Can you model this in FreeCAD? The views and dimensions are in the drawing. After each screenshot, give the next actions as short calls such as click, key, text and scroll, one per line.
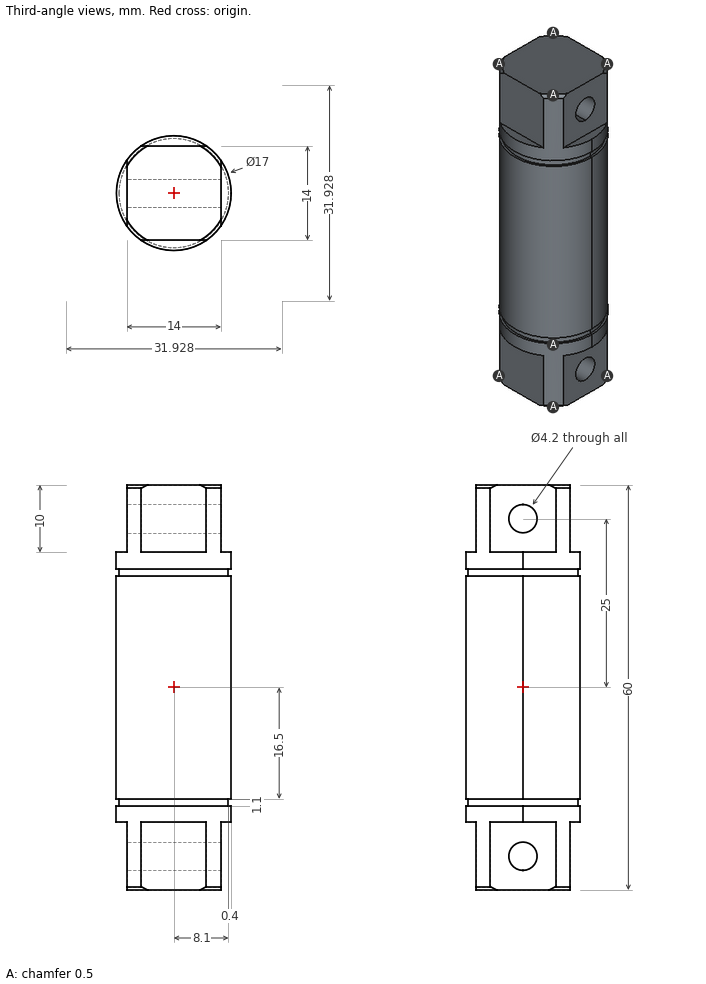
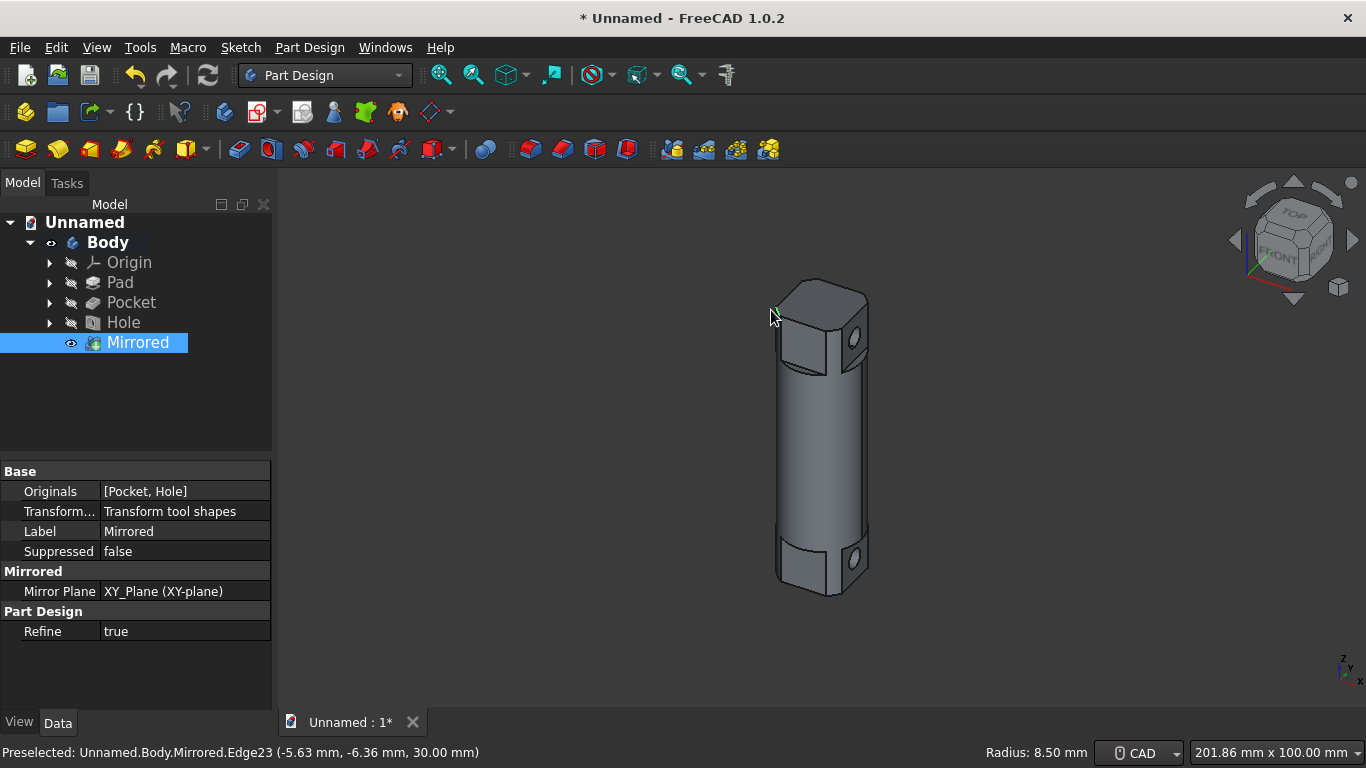
click(834, 329, ctrl)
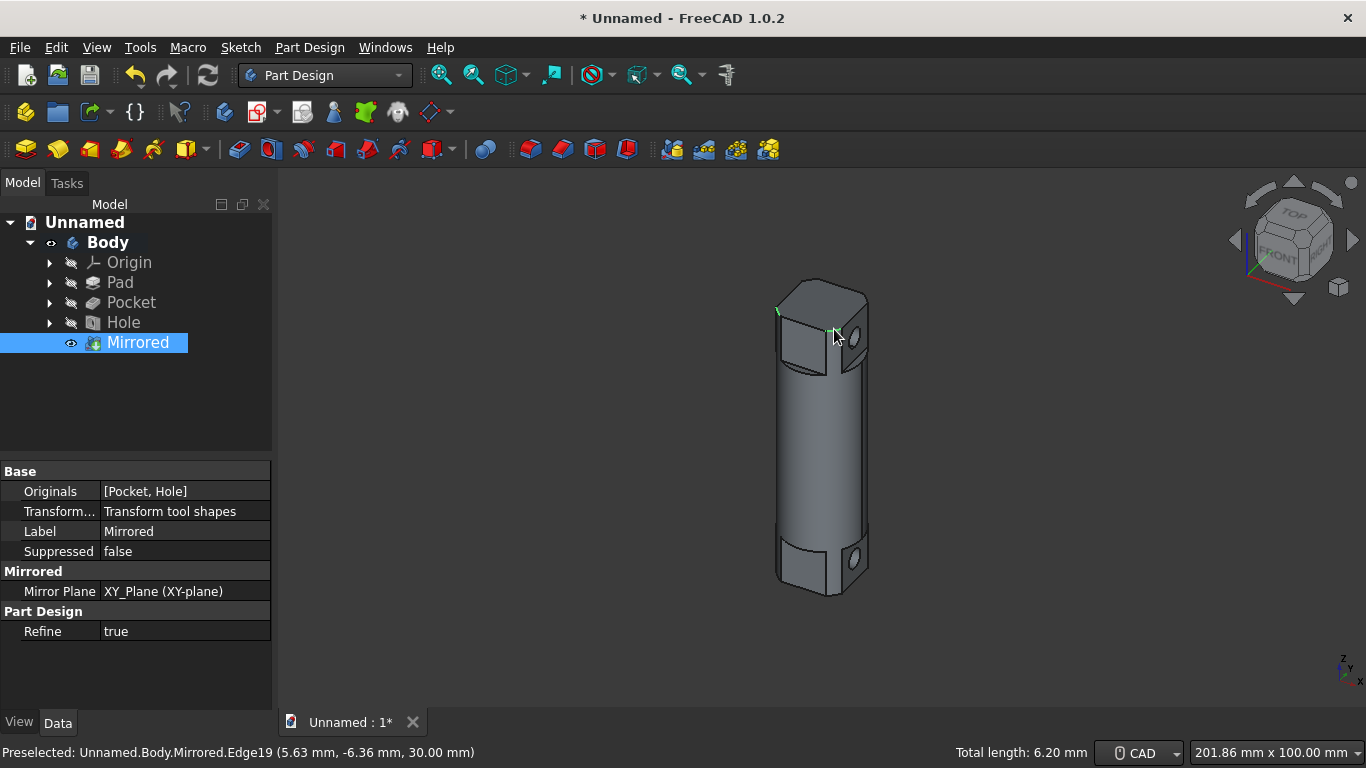
scroll(866, 562, up, 5)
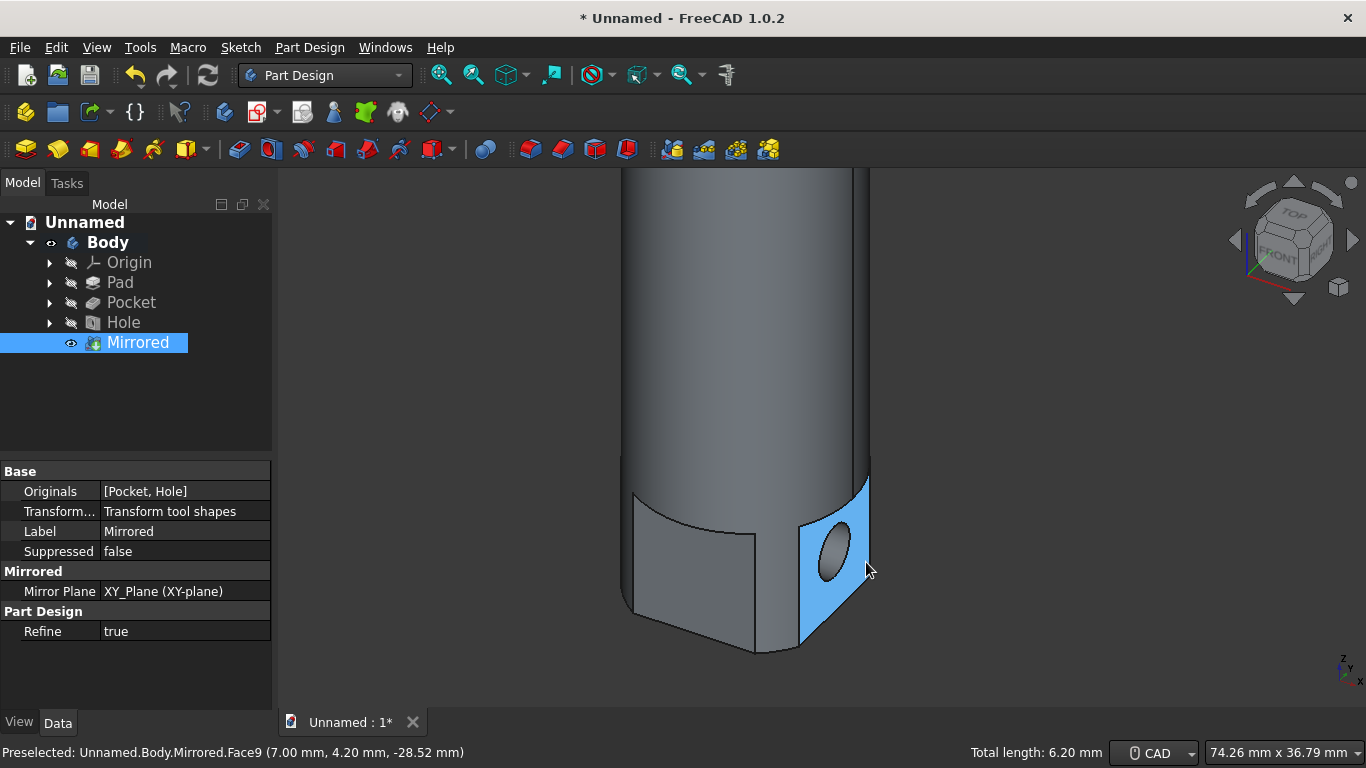
click(442, 76)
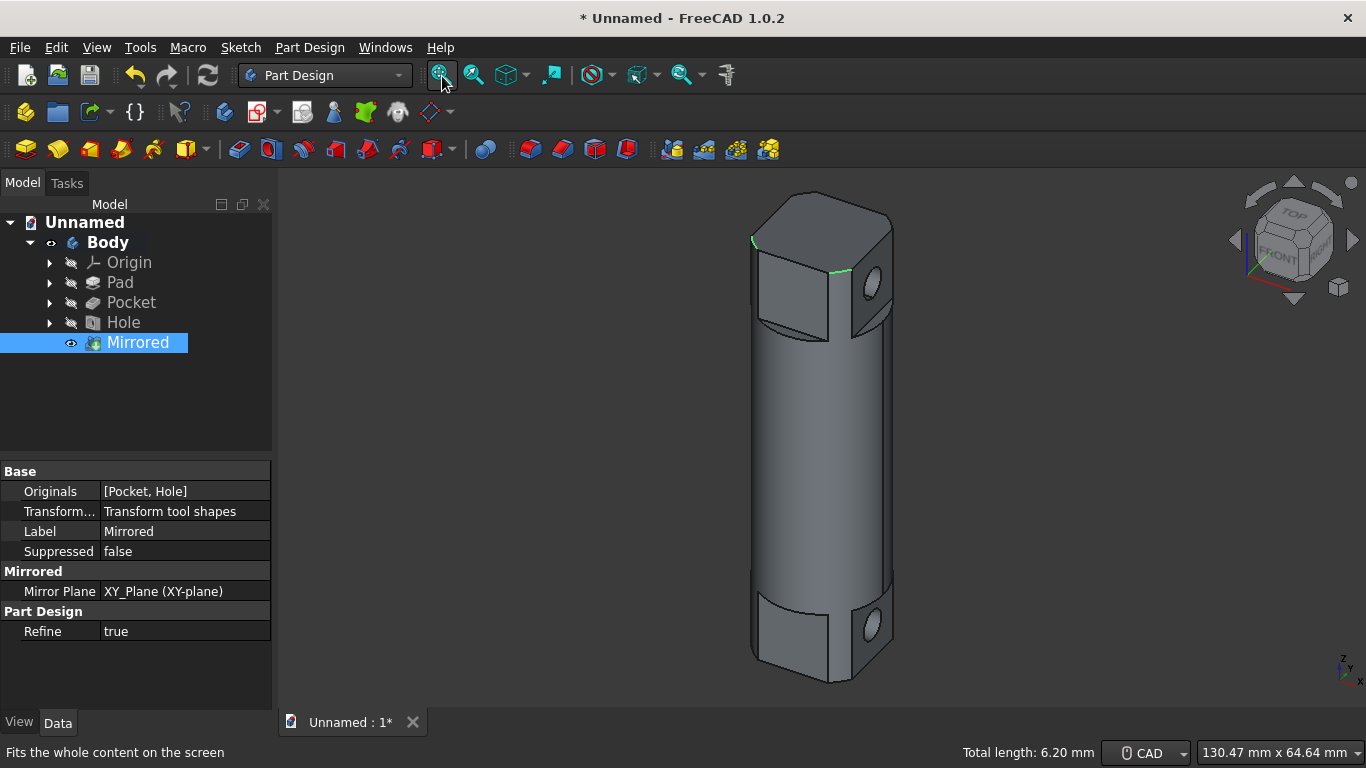
click(891, 222, ctrl)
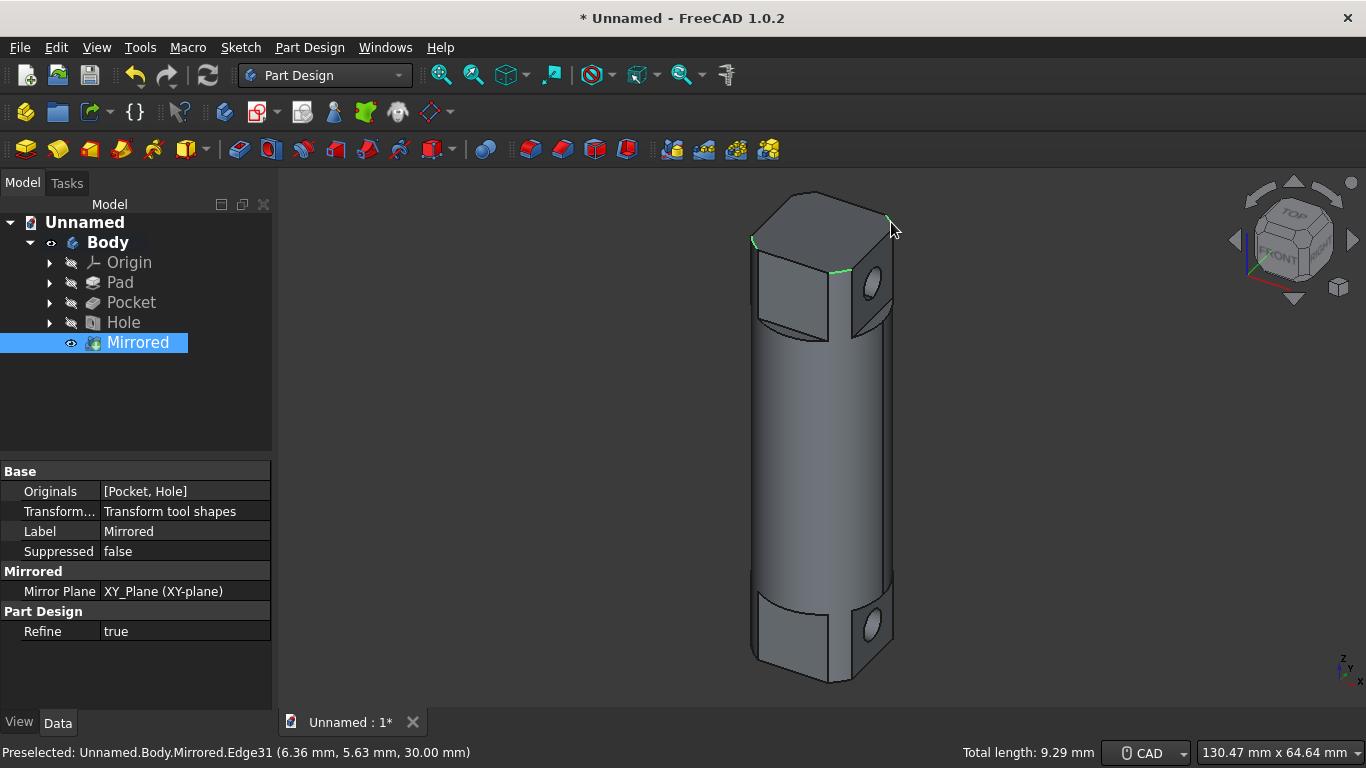
key(v)
key(f)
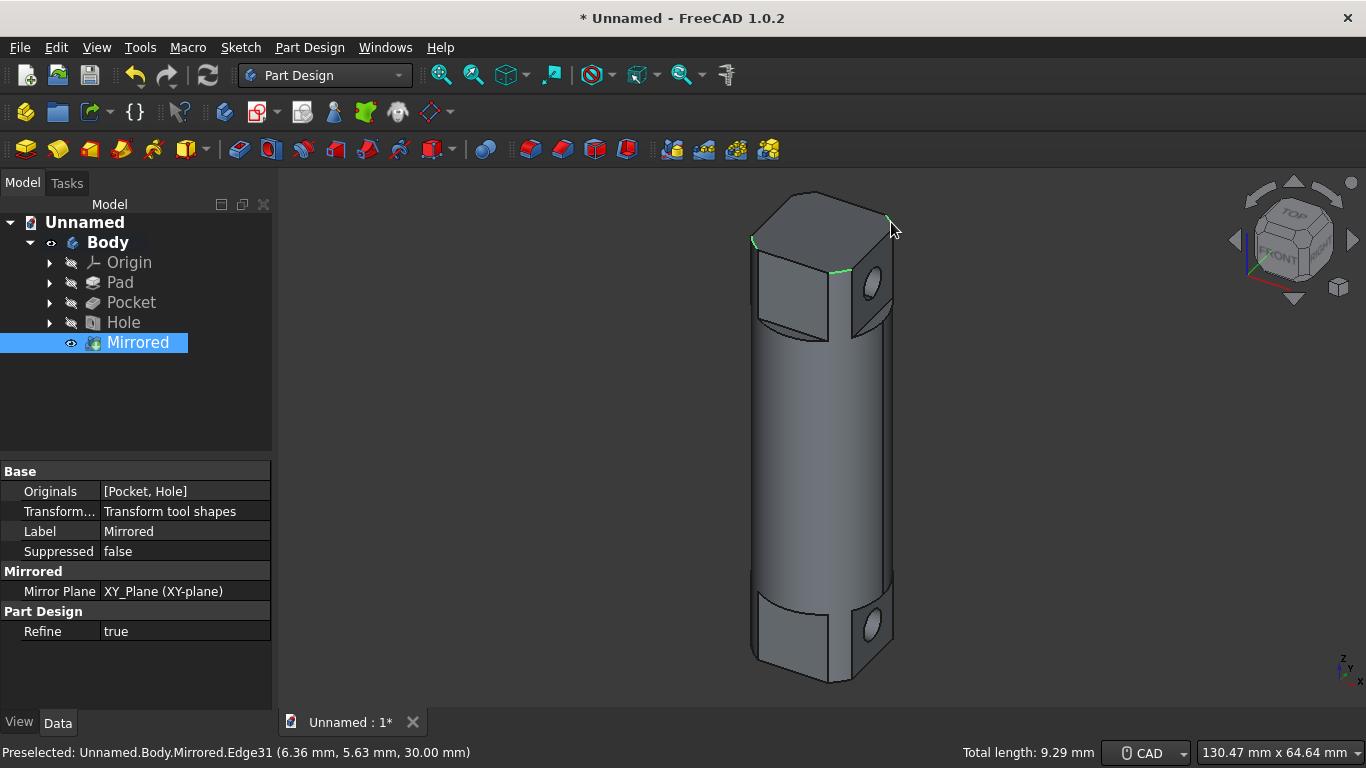
key(0)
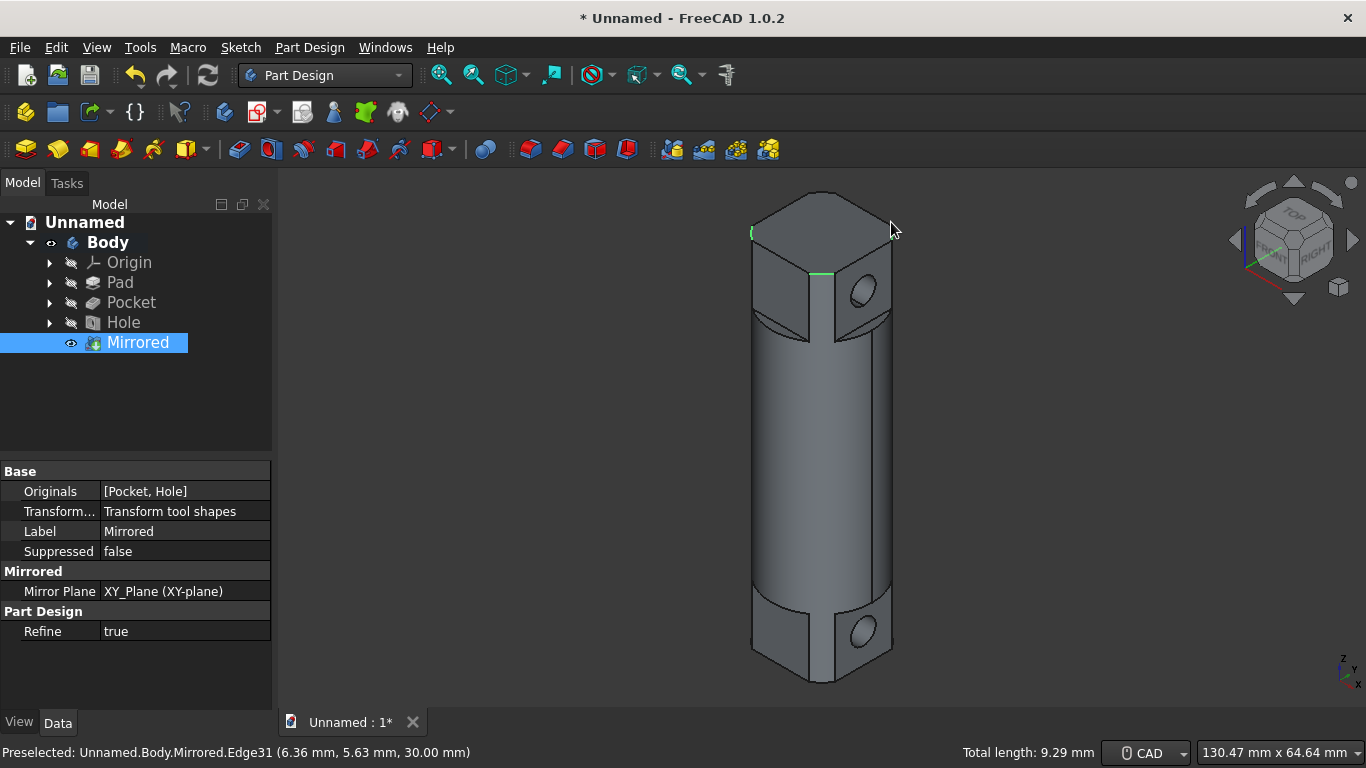
key(2)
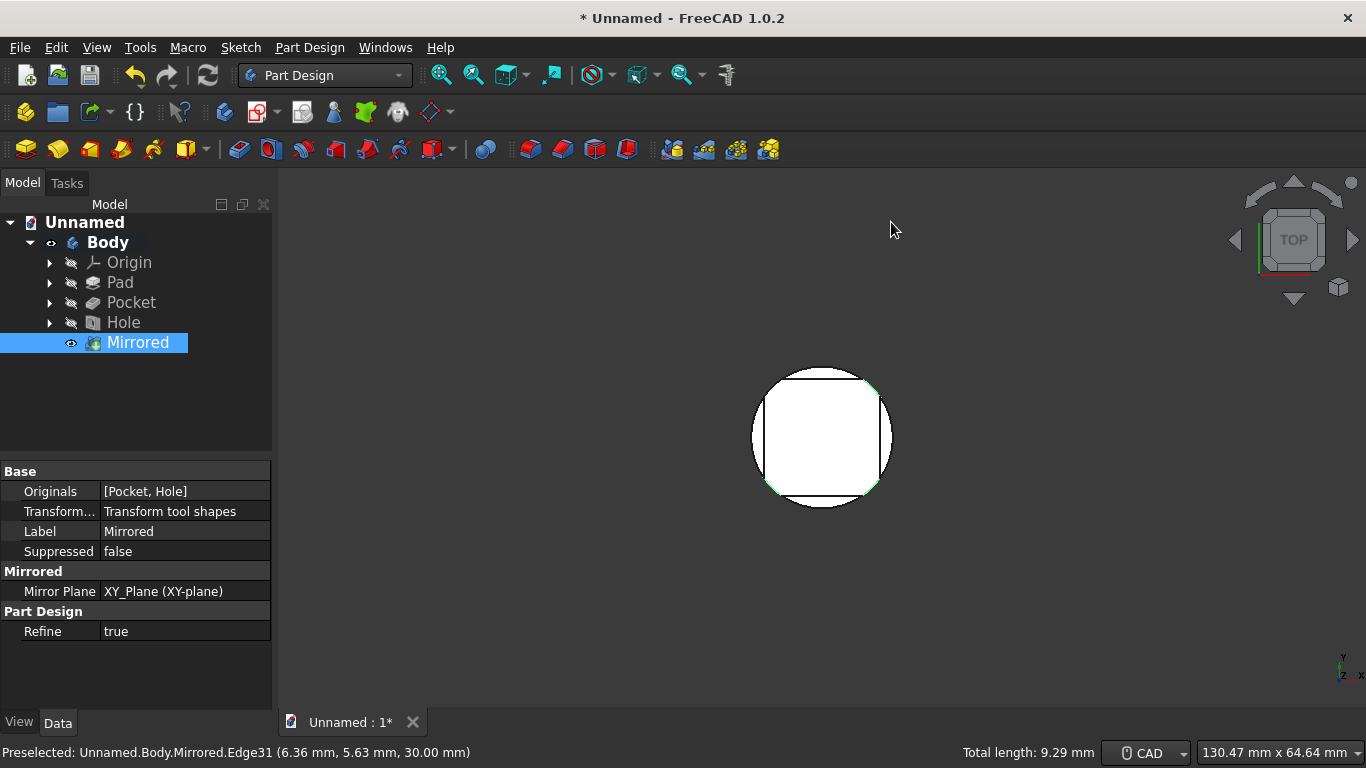
key(v)
key(f)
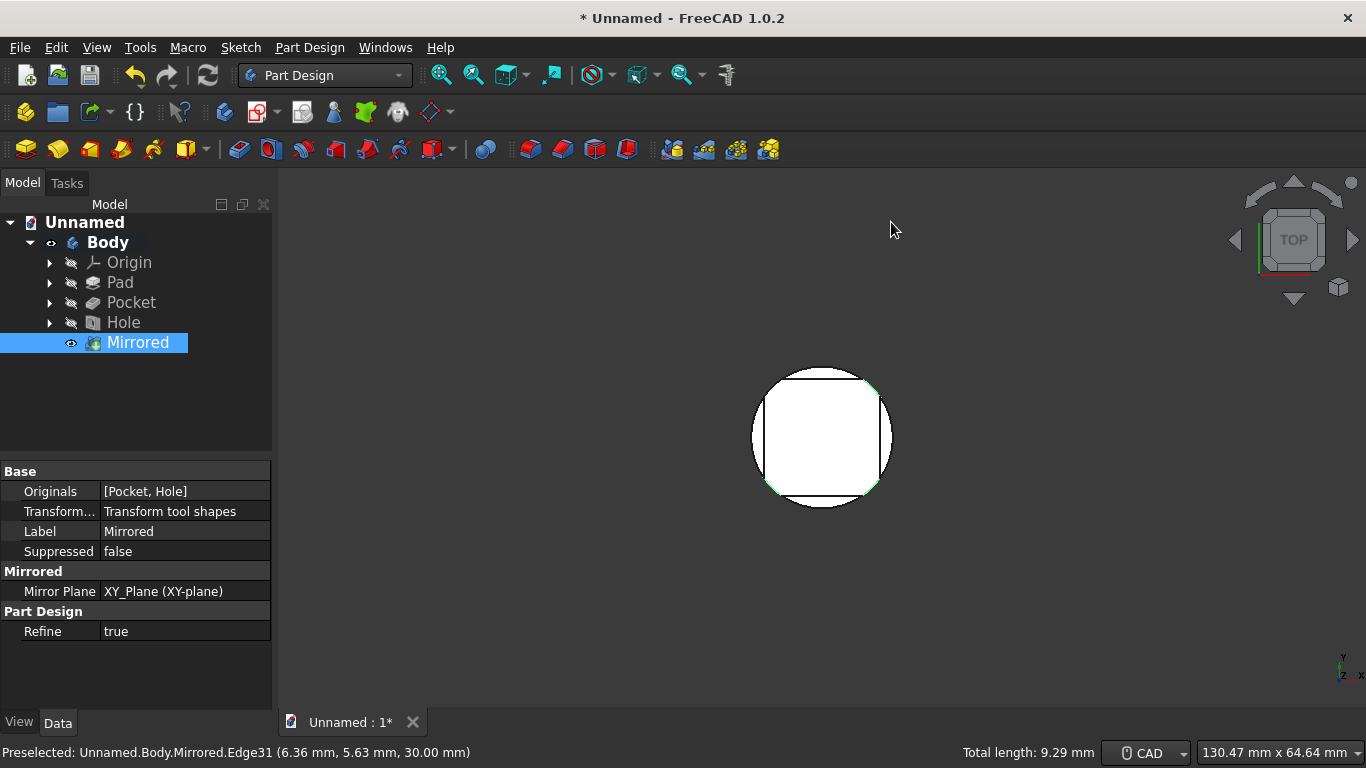
click(772, 386, ctrl)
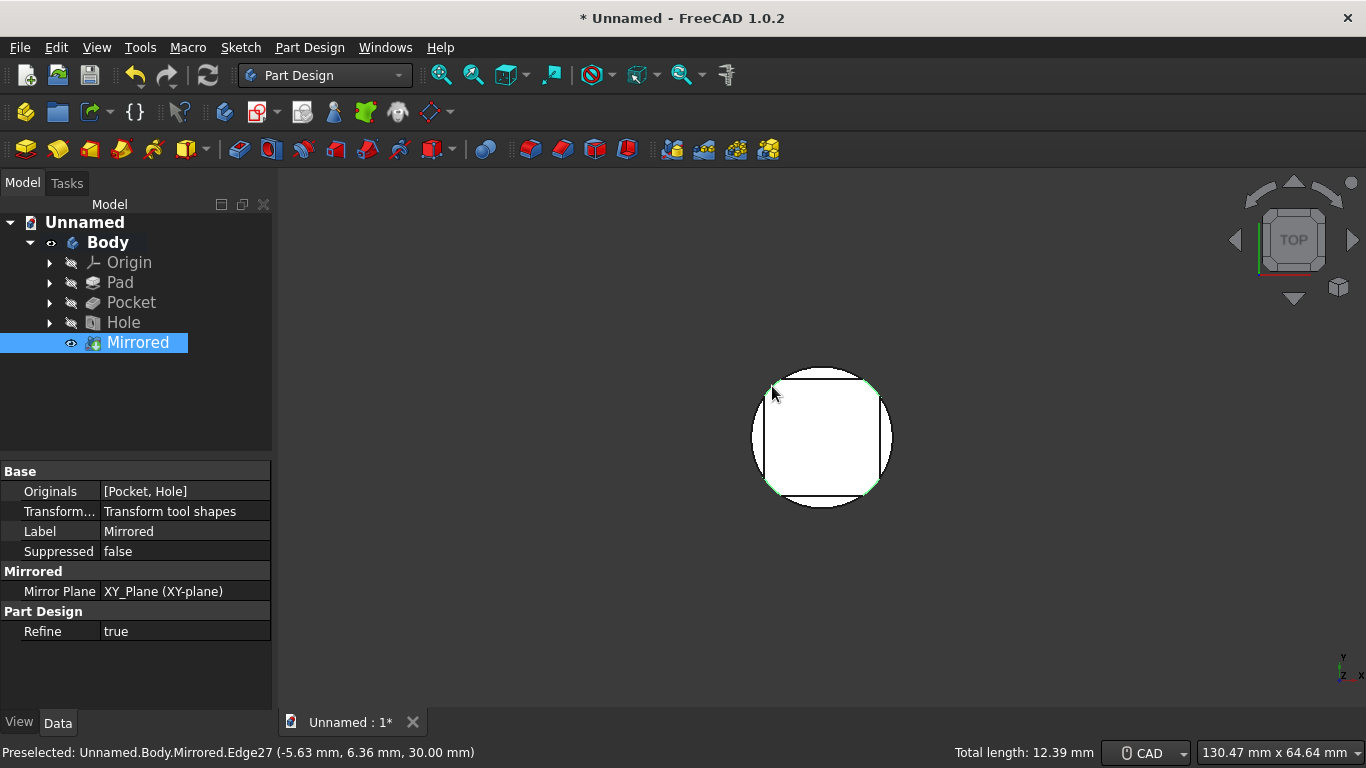
key(1)